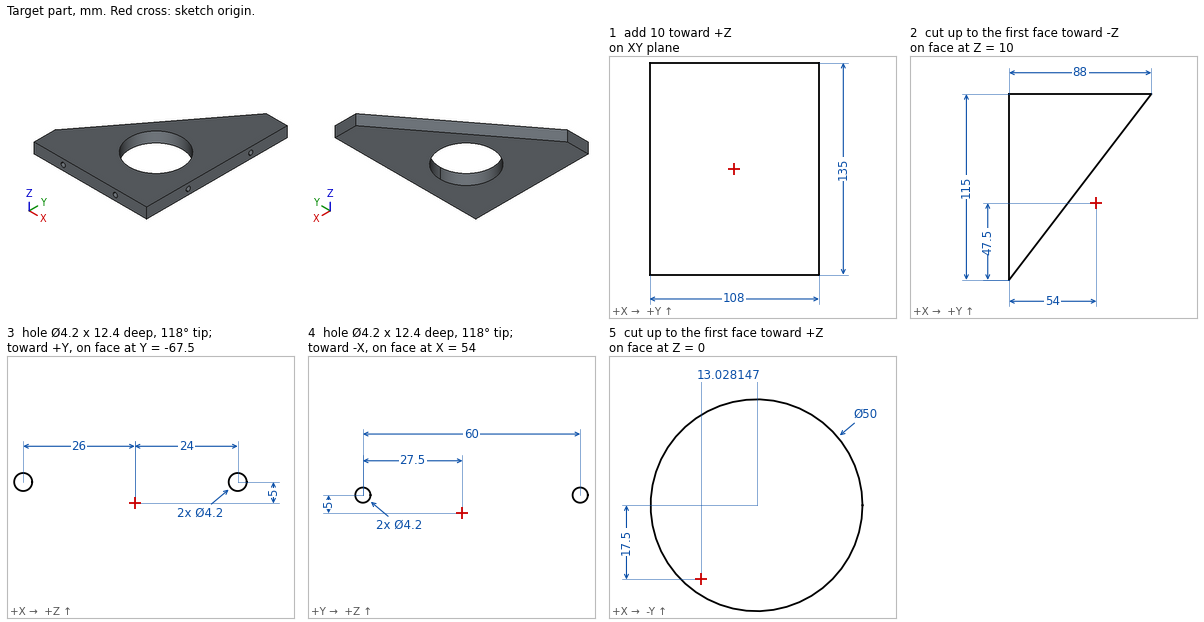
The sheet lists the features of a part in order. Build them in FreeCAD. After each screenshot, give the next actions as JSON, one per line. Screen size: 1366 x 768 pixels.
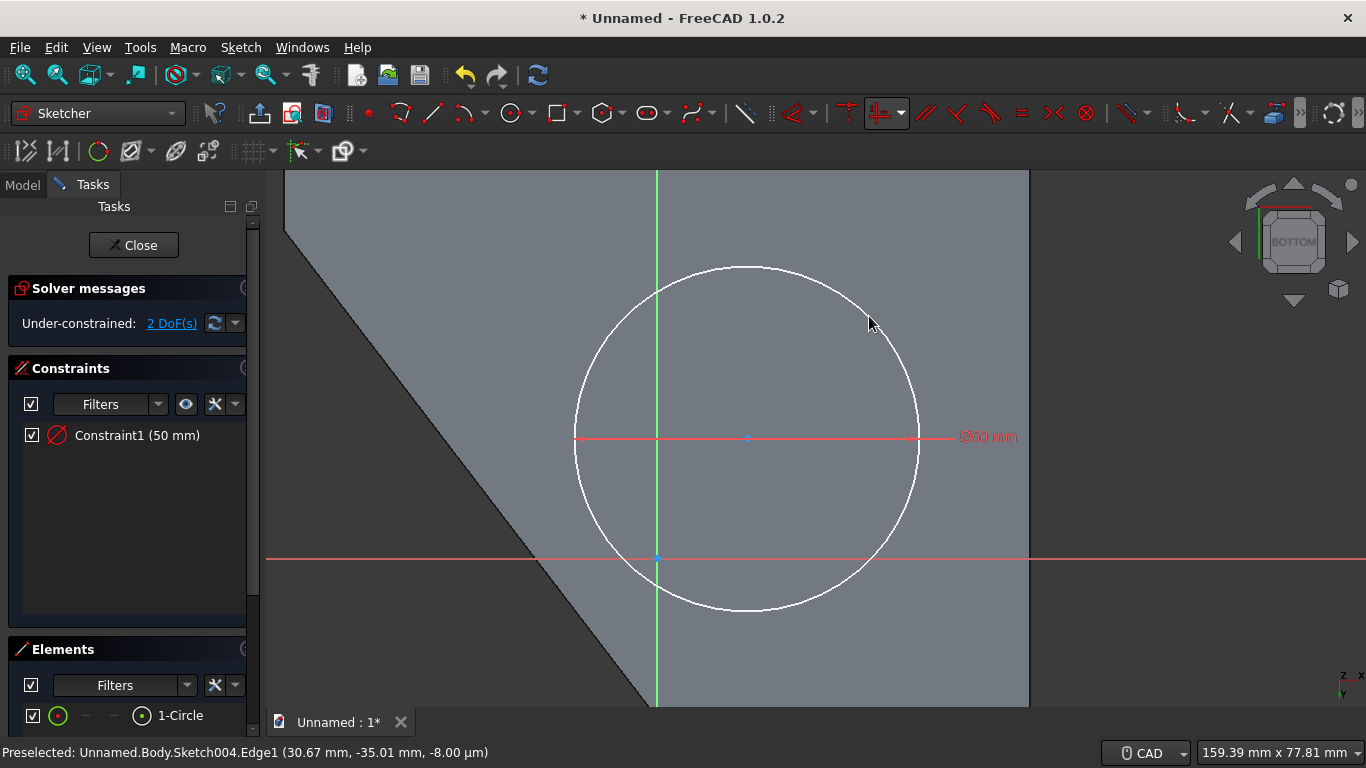
{"action": "key", "text": "d"}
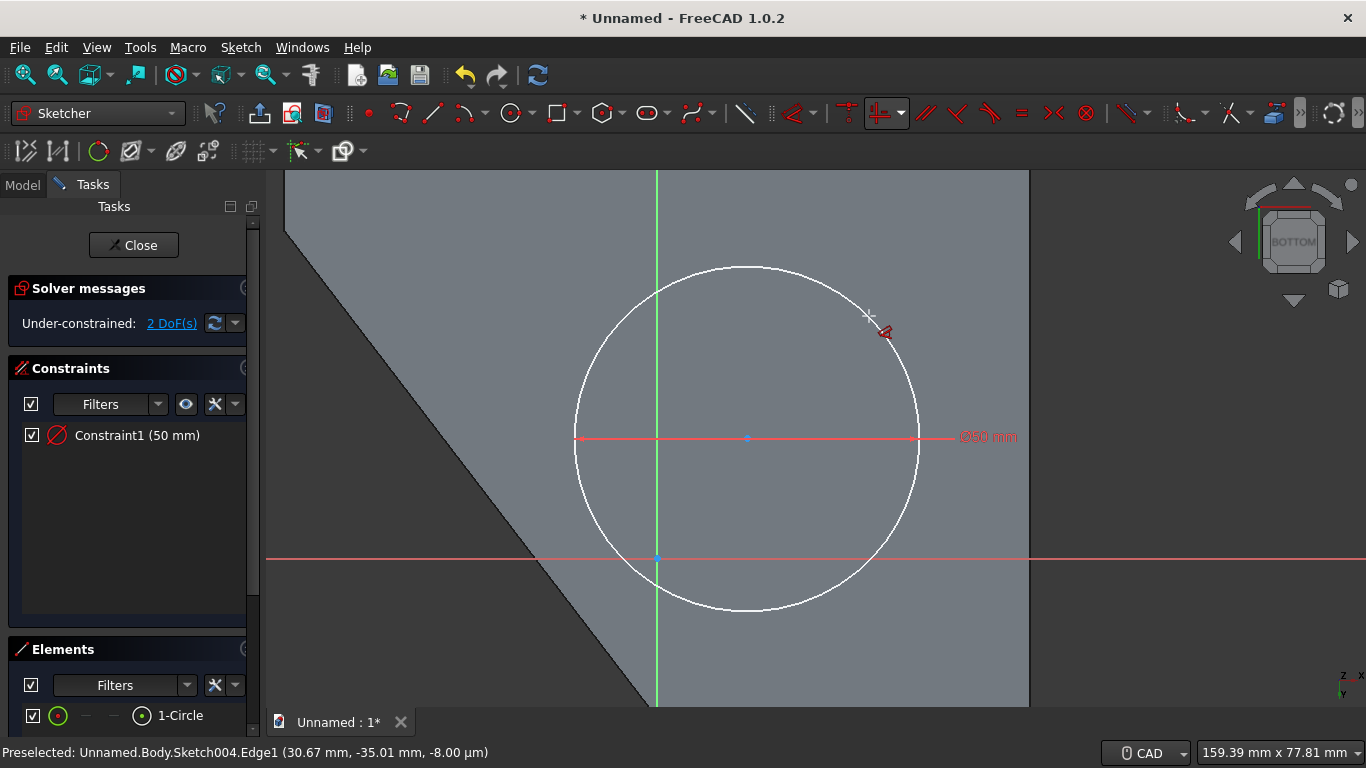
{"action": "left_click", "coordinate": [747, 439]}
{"action": "left_click", "coordinate": [623, 499]}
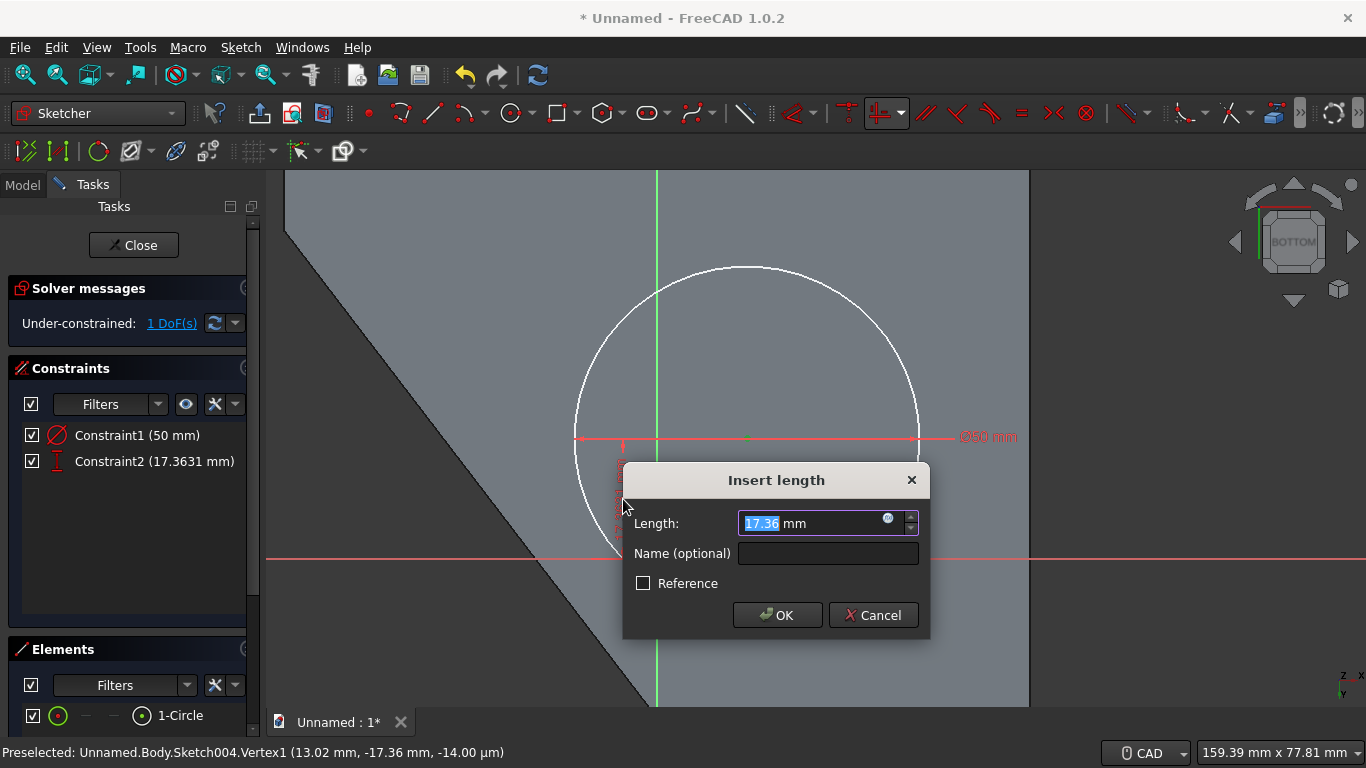
{"action": "type", "text": "17.5"}
{"action": "key", "text": "Return"}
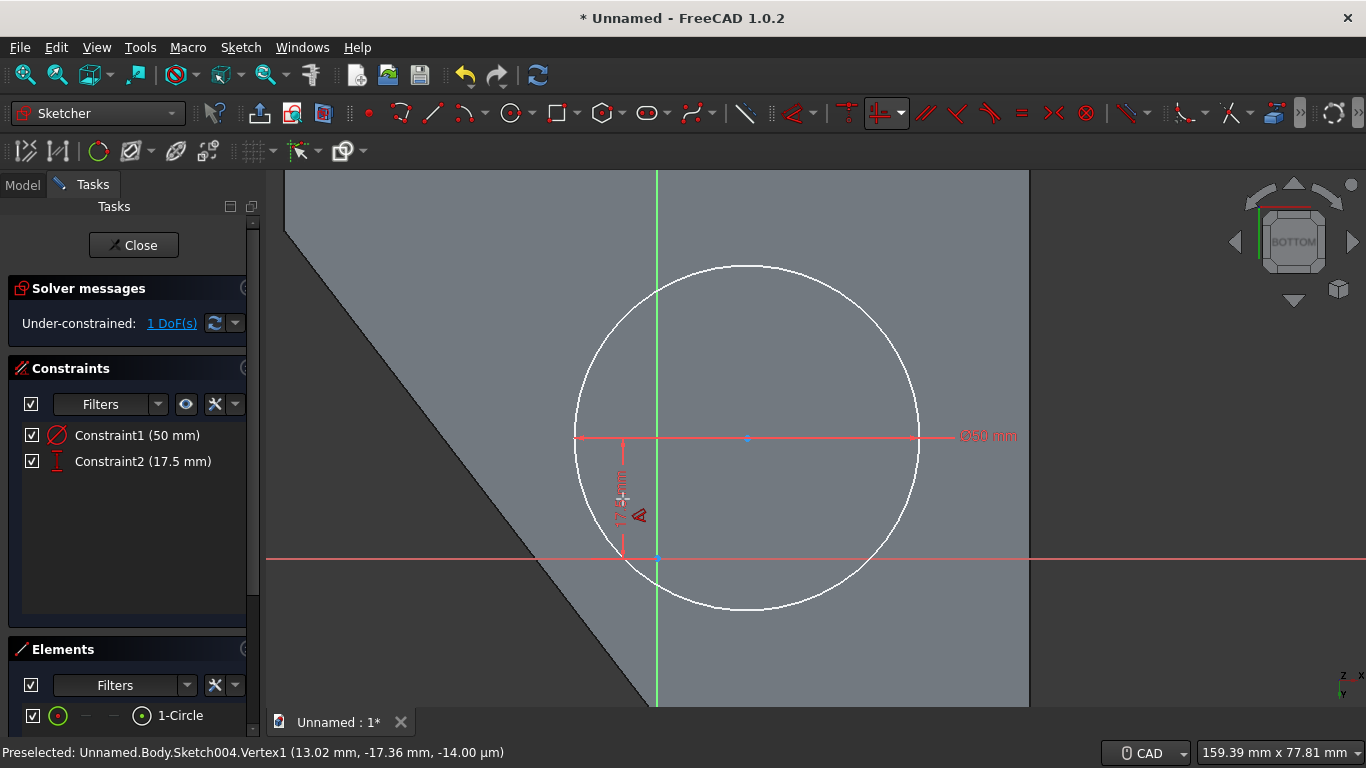
{"action": "left_click", "coordinate": [747, 438]}
{"action": "left_click", "coordinate": [723, 593]}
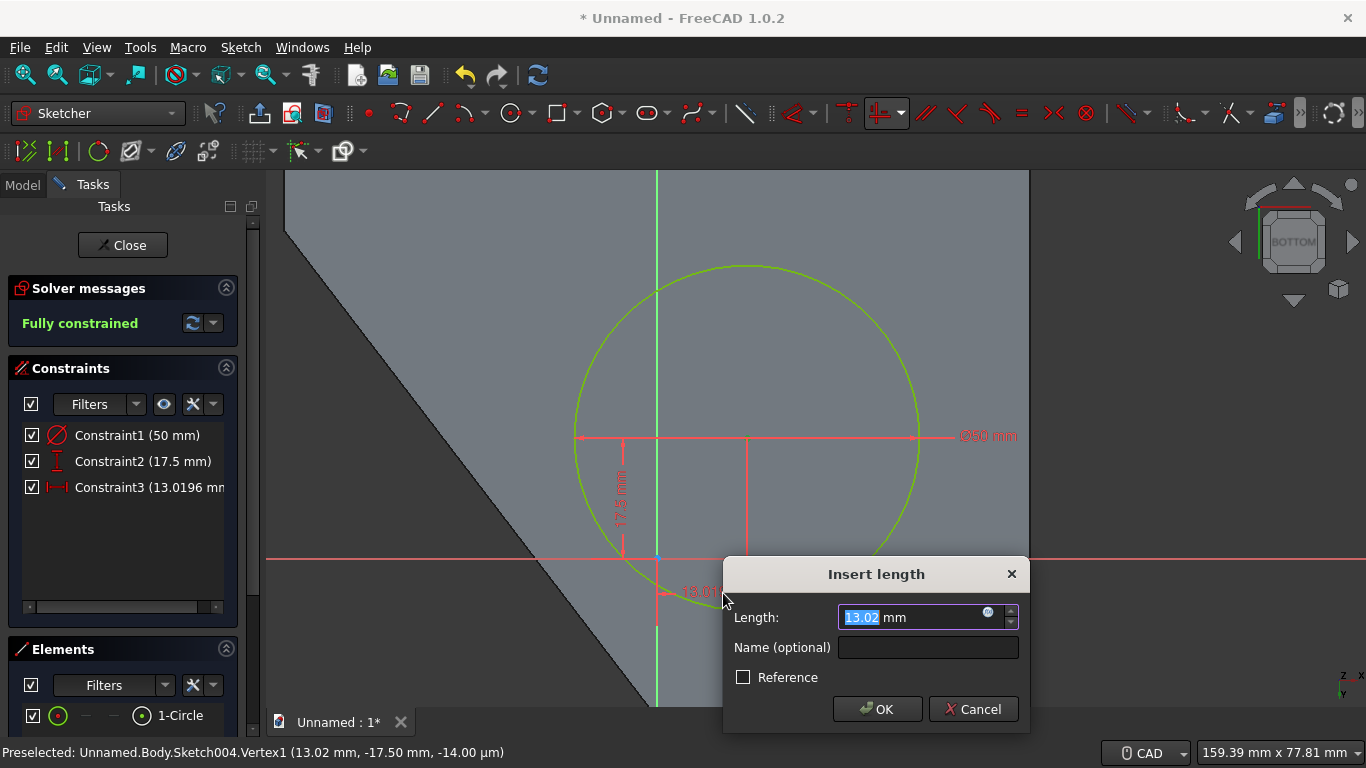
{"action": "type", "text": "13.028147"}
{"action": "key", "text": "Return"}
{"action": "key", "text": "Escape"}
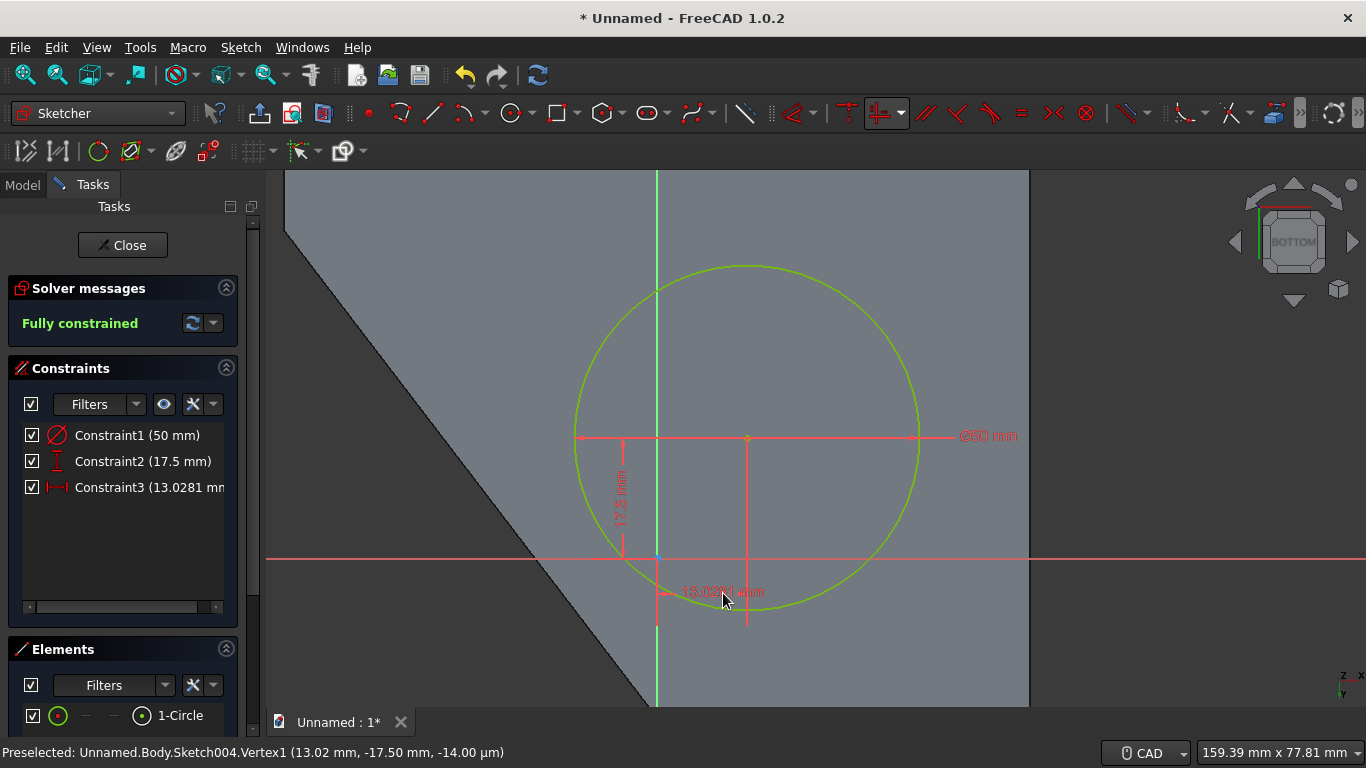
{"action": "left_click", "coordinate": [123, 245]}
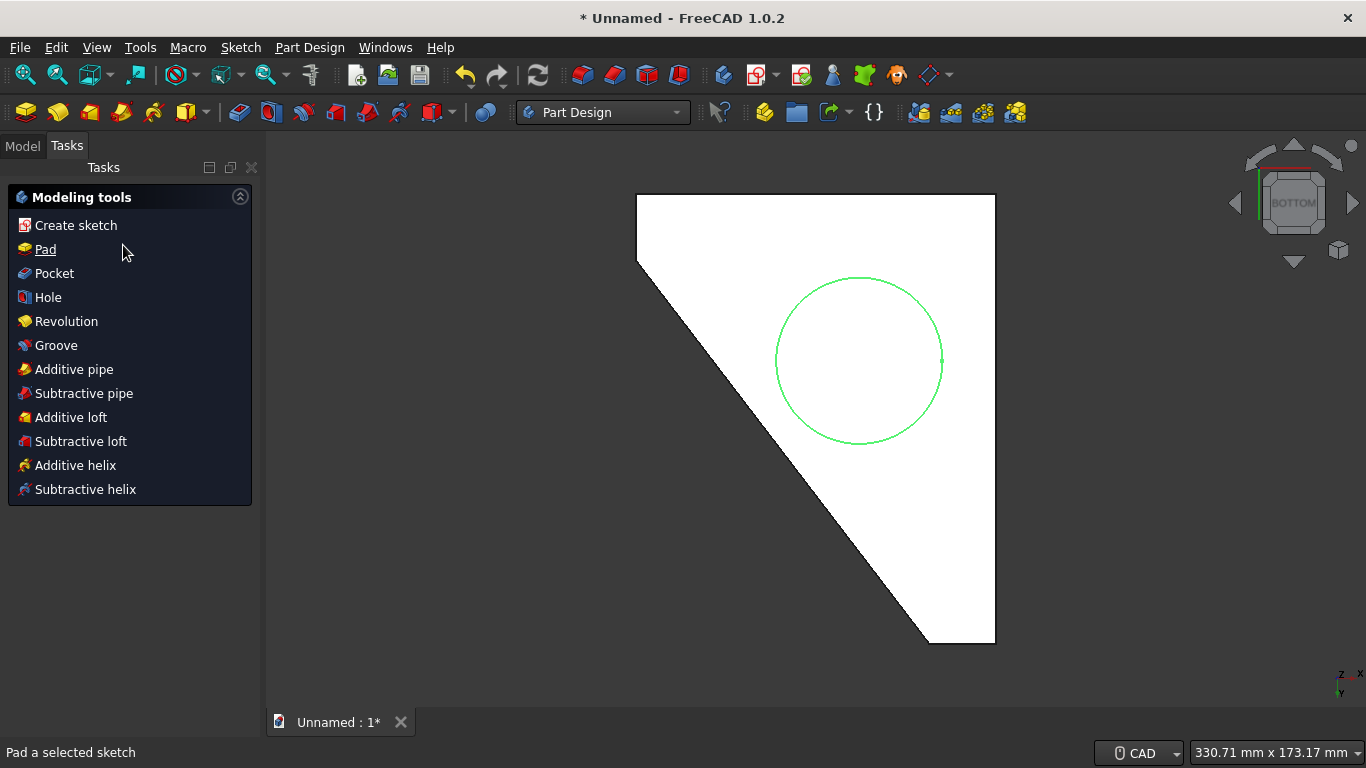
{"action": "left_click", "coordinate": [240, 112]}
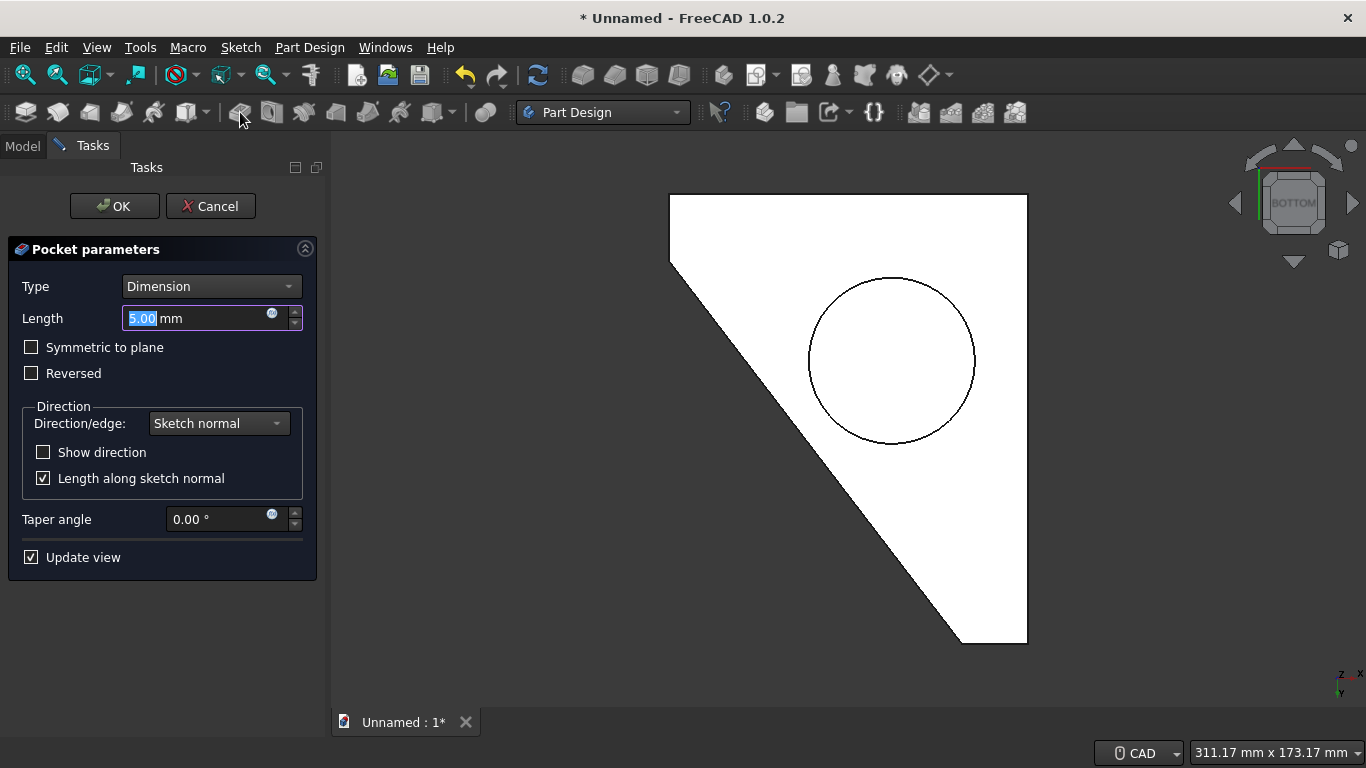
{"action": "left_click", "coordinate": [212, 286]}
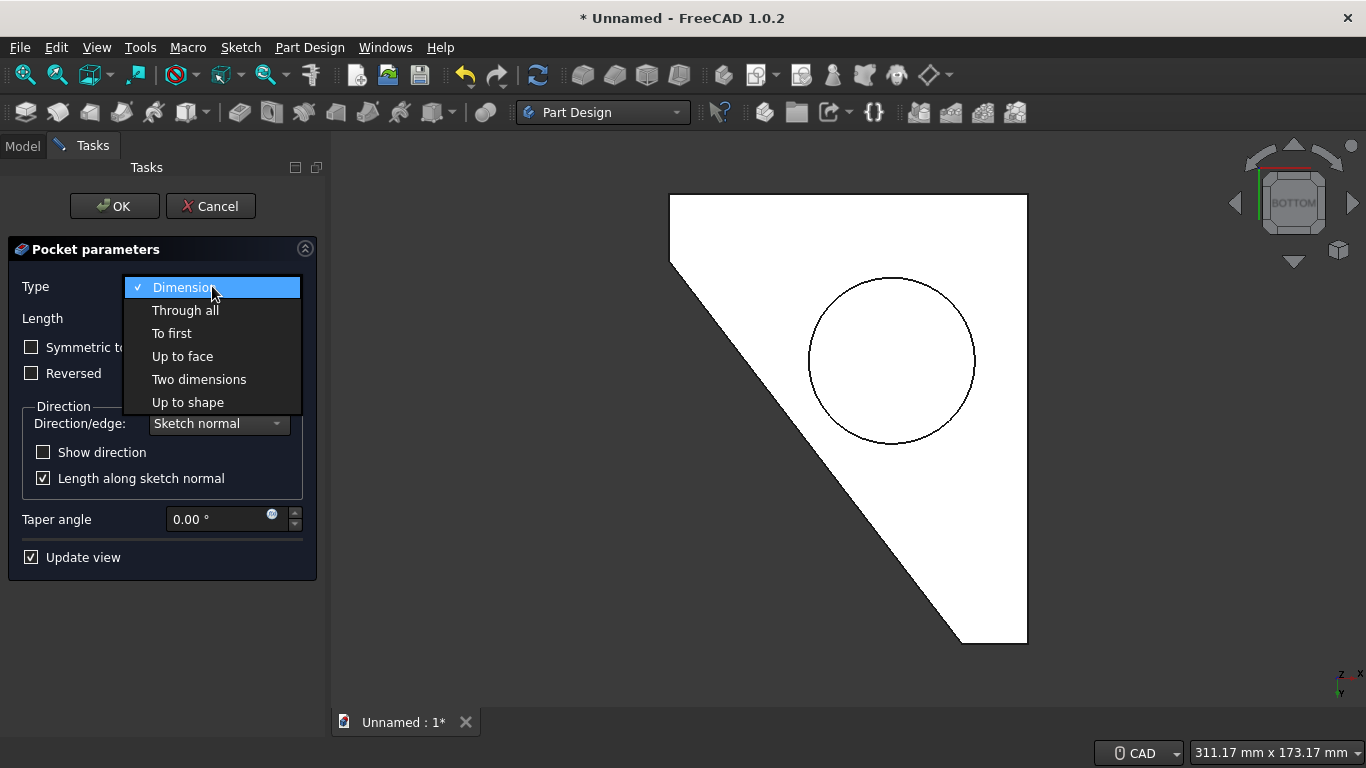
{"action": "left_click", "coordinate": [212, 334]}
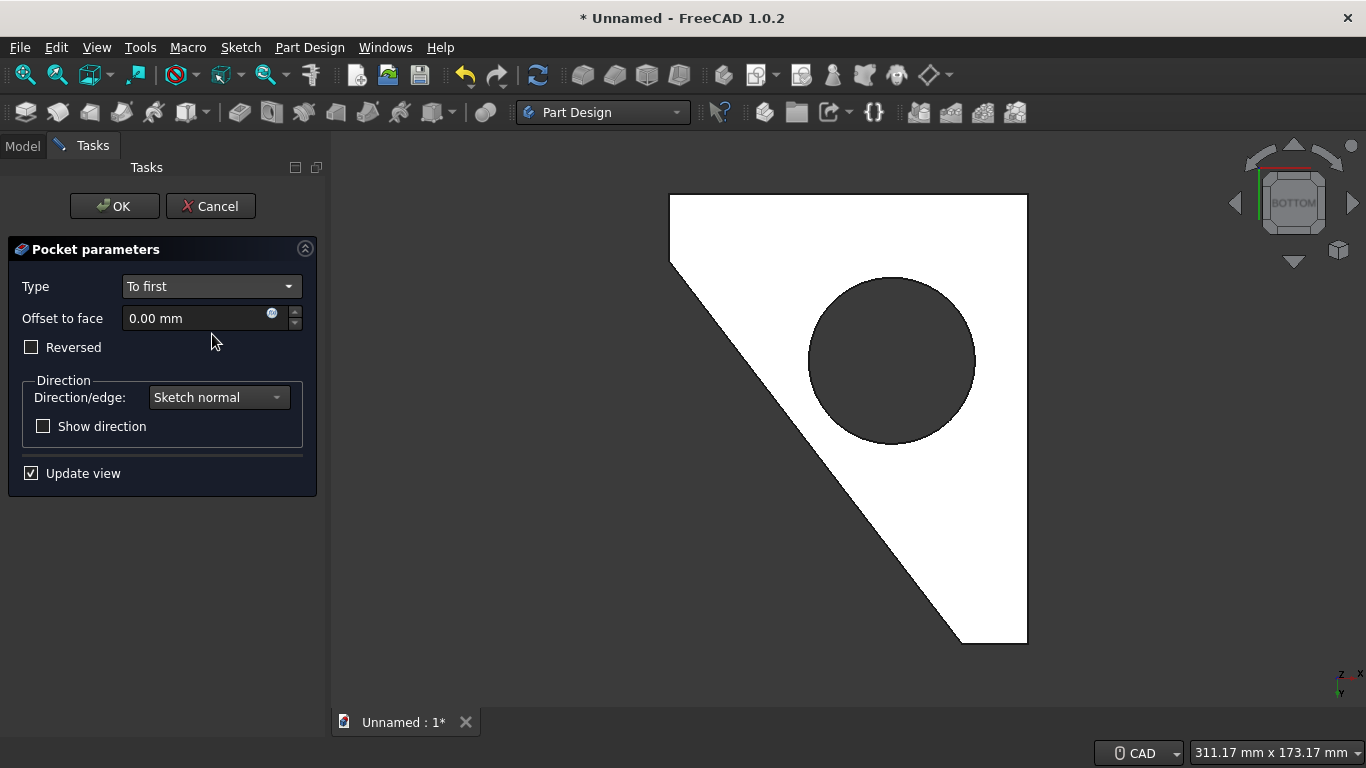
{"action": "left_click", "coordinate": [115, 206]}